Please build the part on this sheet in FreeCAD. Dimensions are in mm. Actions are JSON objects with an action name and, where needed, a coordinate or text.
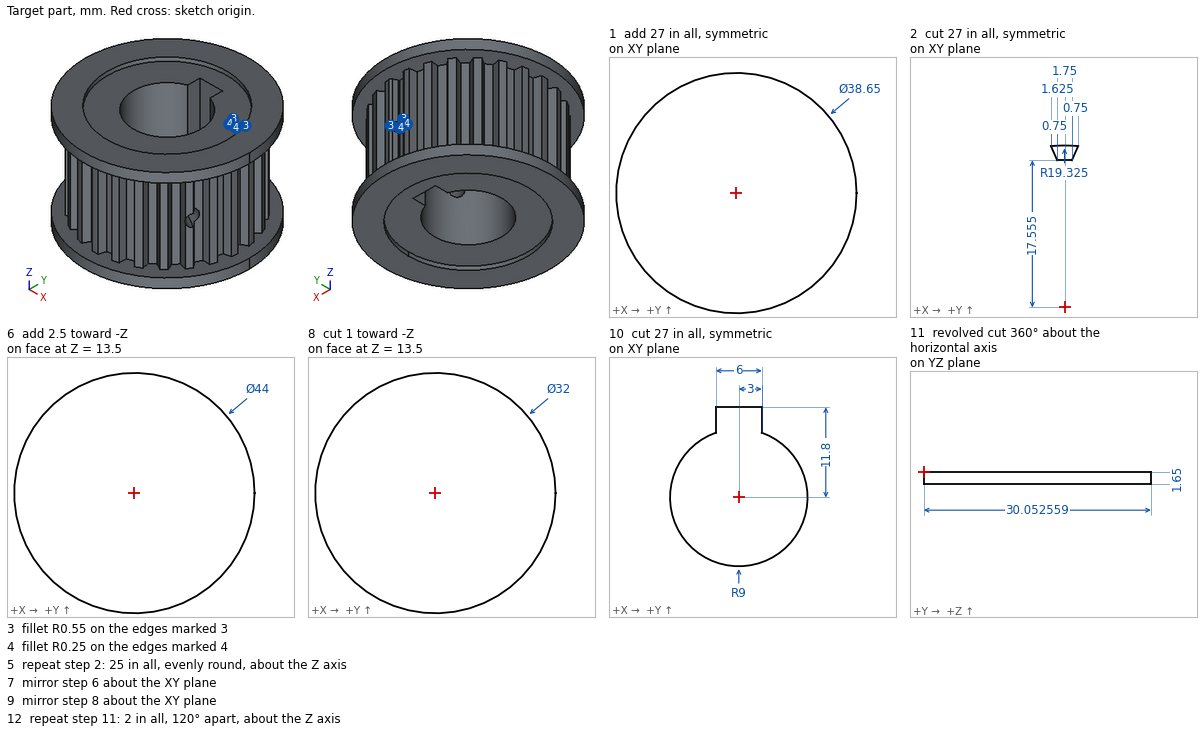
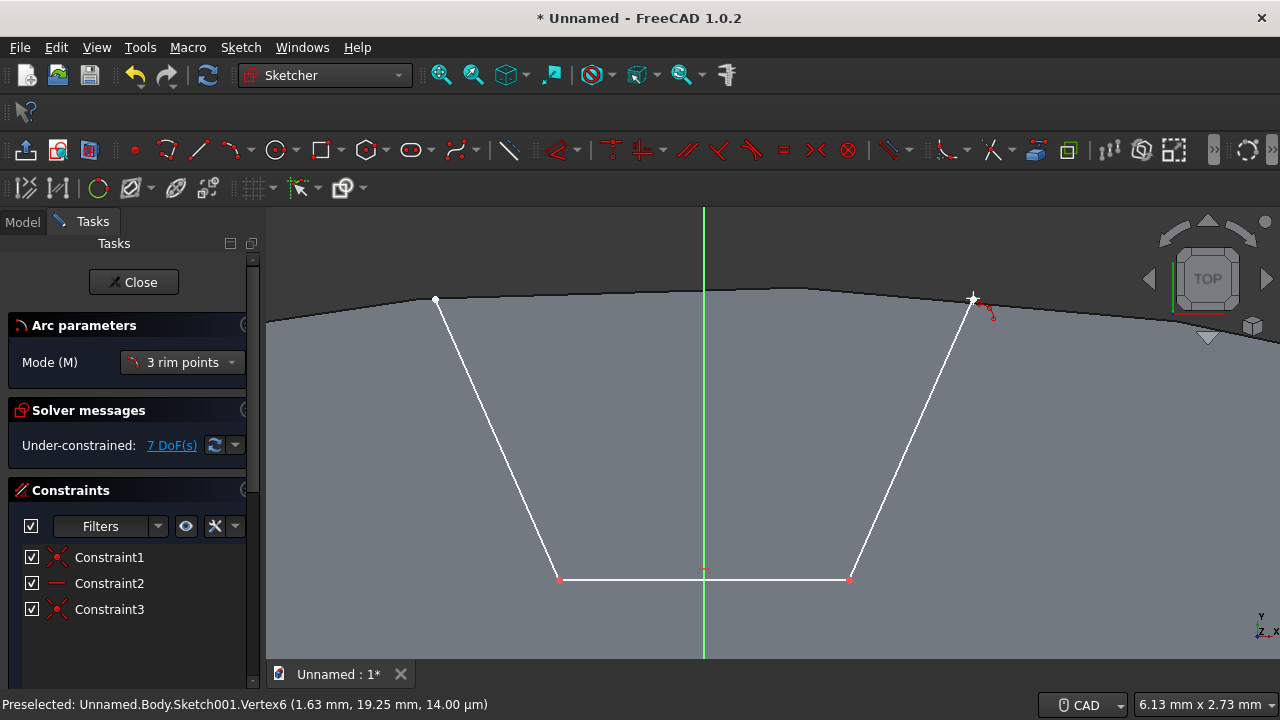
{"action": "left_click", "coordinate": [973, 299]}
{"action": "left_click", "coordinate": [435, 299]}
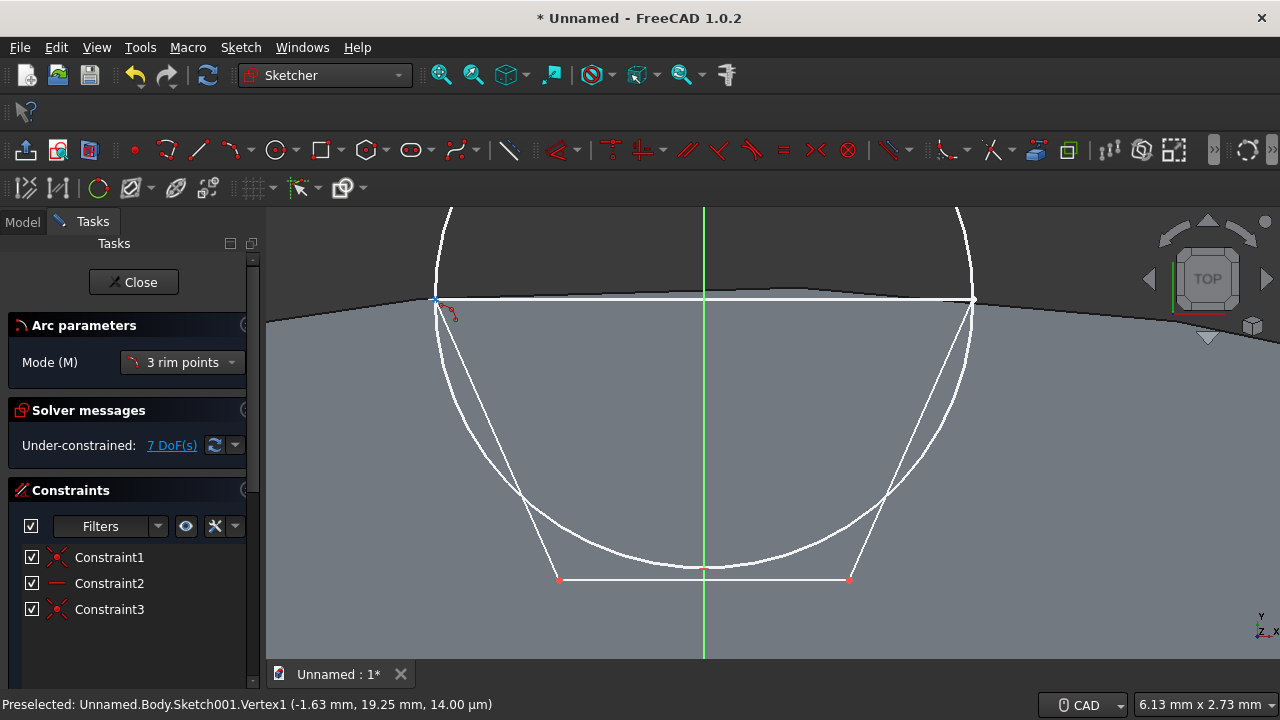
{"action": "scroll", "coordinate": [758, 287], "scroll_direction": "up", "scroll_amount": 2}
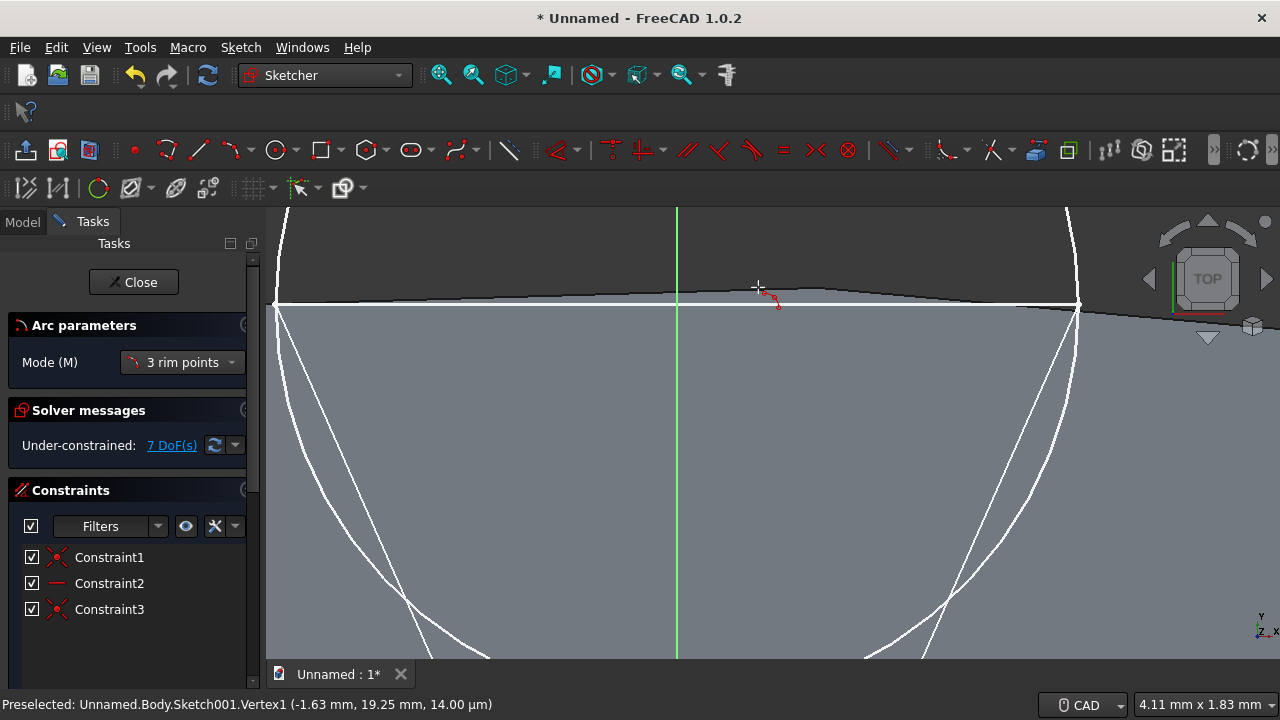
{"action": "left_click", "coordinate": [757, 286]}
{"action": "key", "text": "Escape"}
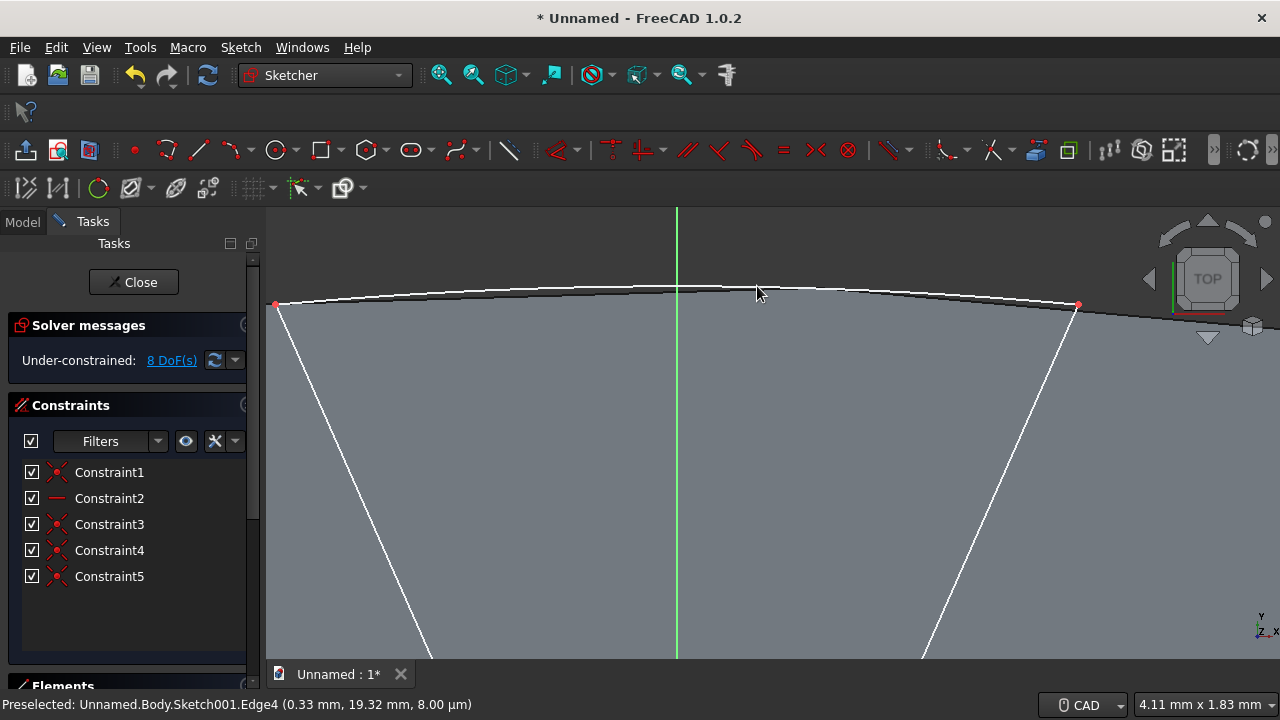
{"action": "scroll", "coordinate": [760, 288], "scroll_direction": "down", "scroll_amount": 2}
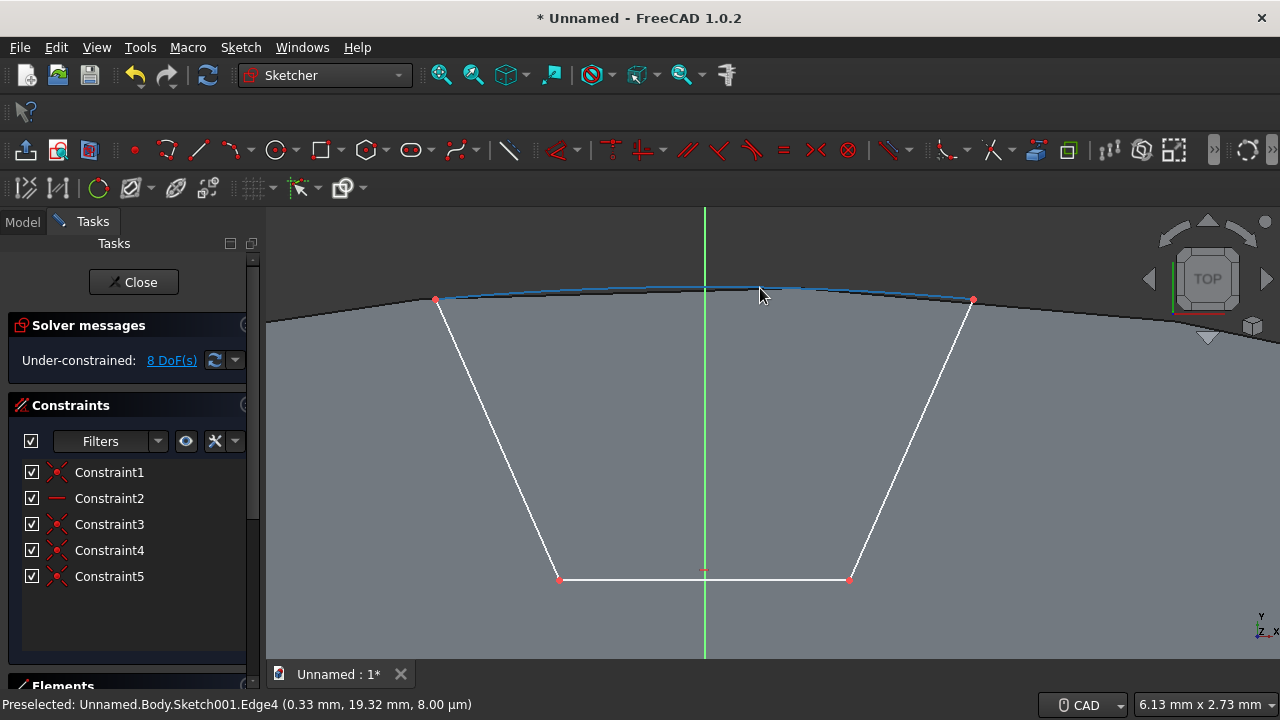
{"action": "scroll", "coordinate": [704, 295], "scroll_direction": "down", "scroll_amount": 12}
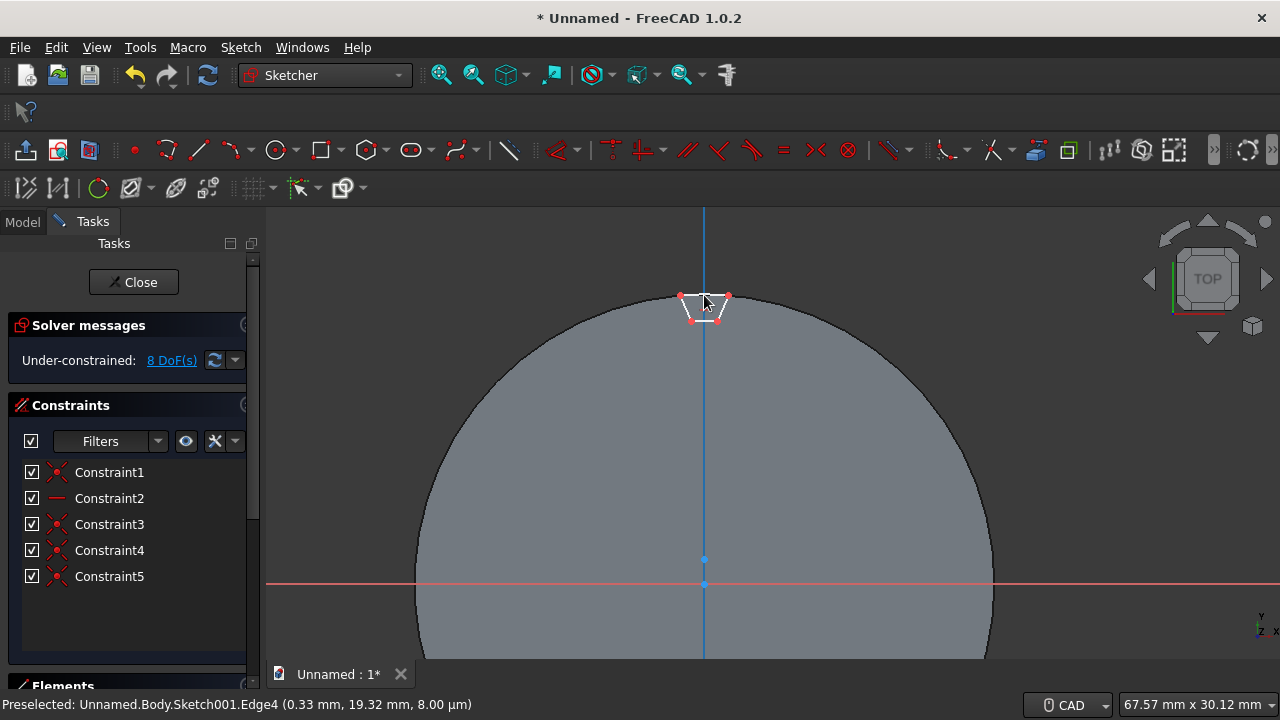
{"action": "left_click_drag", "start_coordinate": [694, 549], "coordinate": [714, 594]}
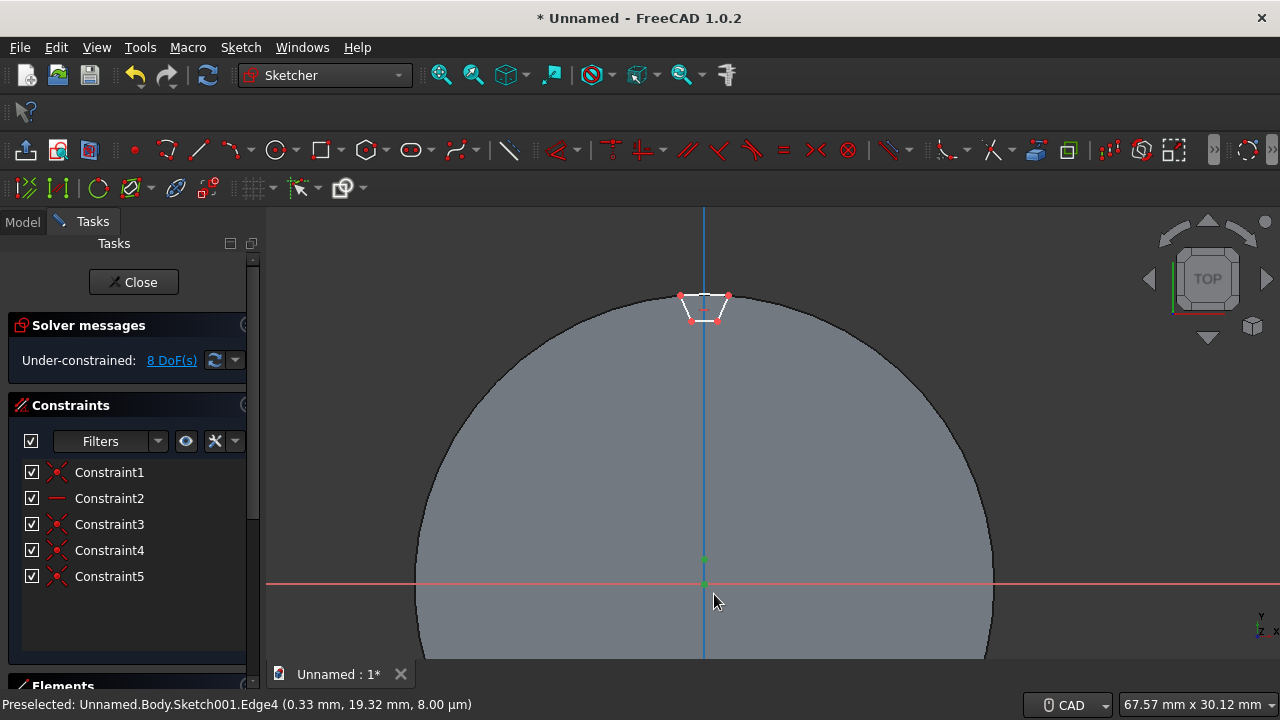
{"action": "left_click", "coordinate": [612, 150]}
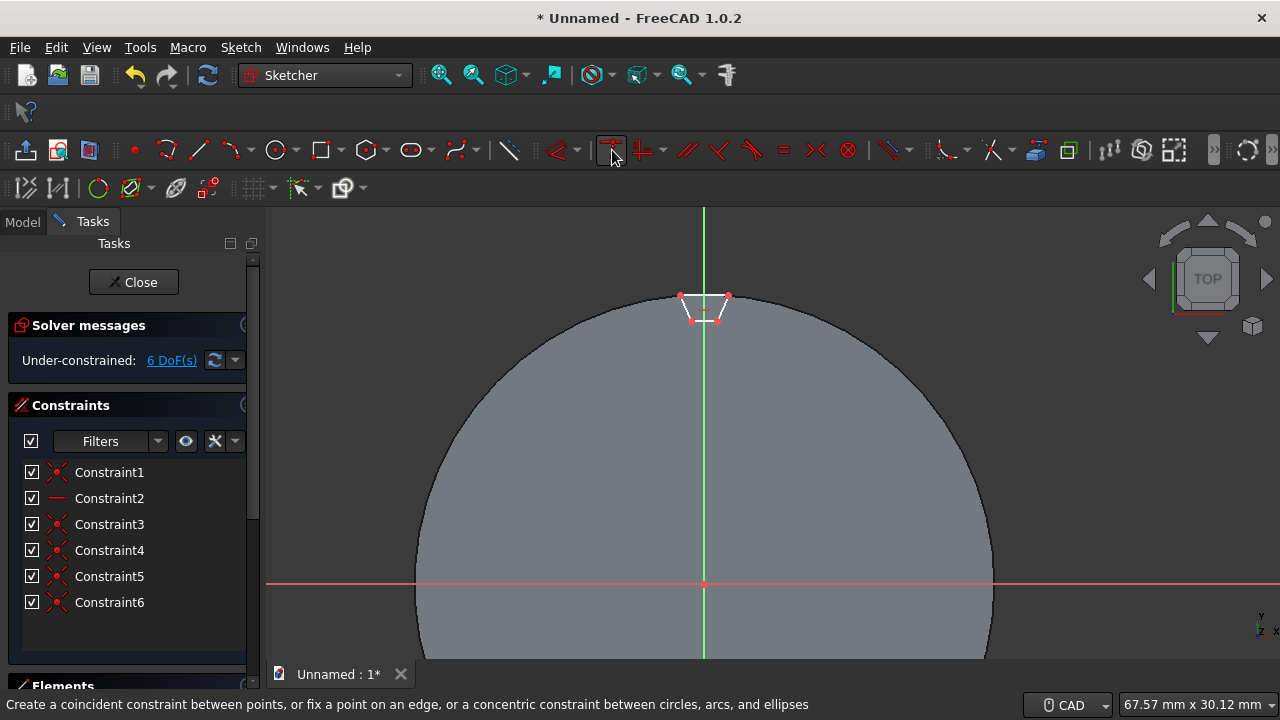
{"action": "scroll", "coordinate": [714, 295], "scroll_direction": "up", "scroll_amount": 2}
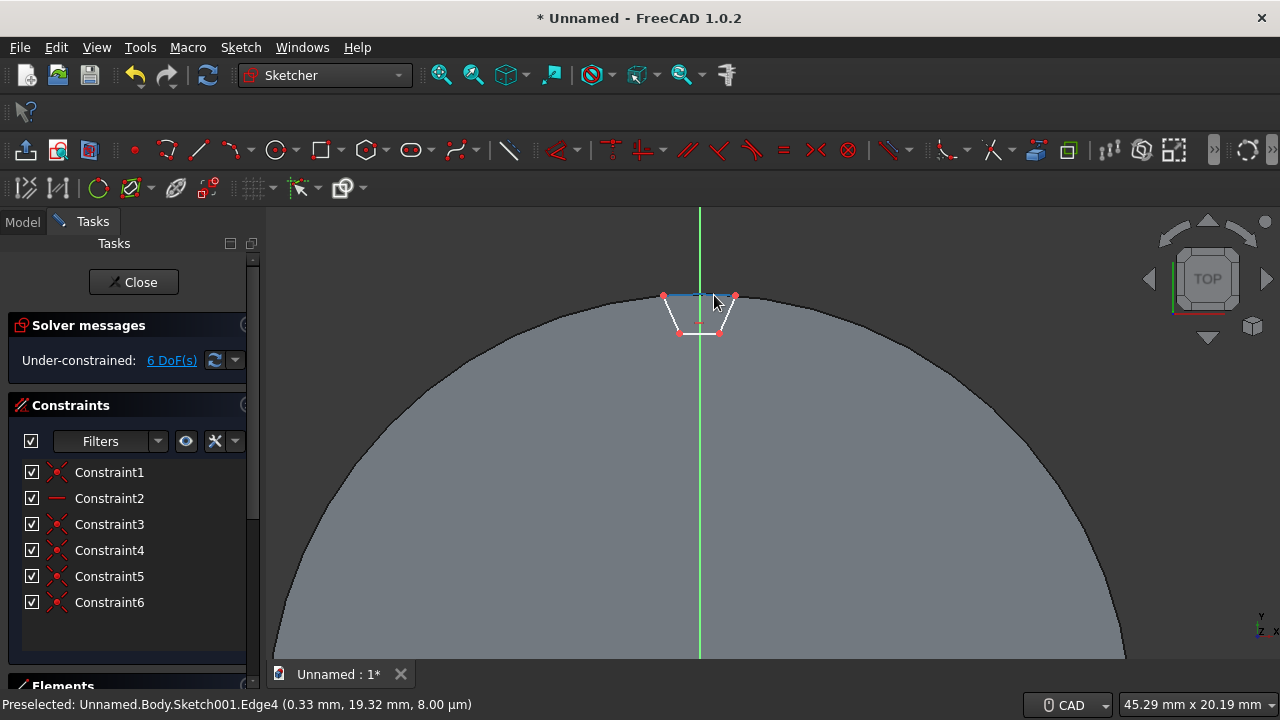
{"action": "left_click", "coordinate": [714, 295]}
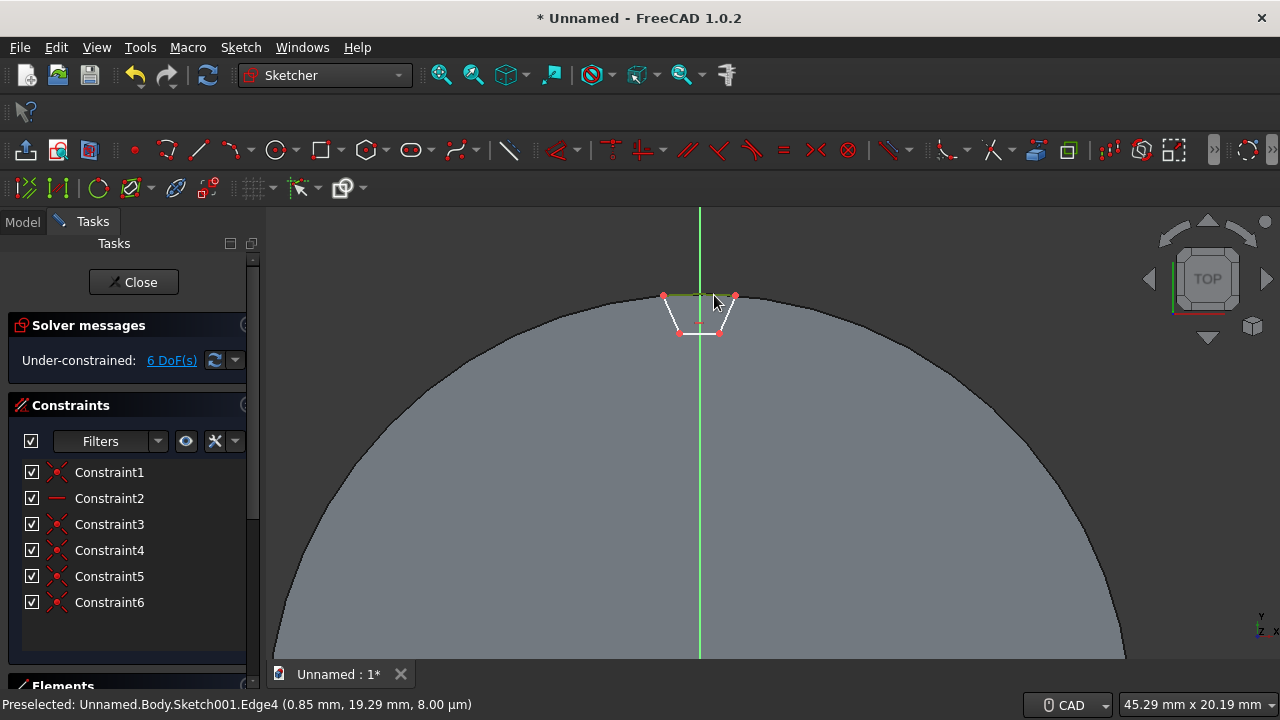
{"action": "left_click", "coordinate": [580, 150]}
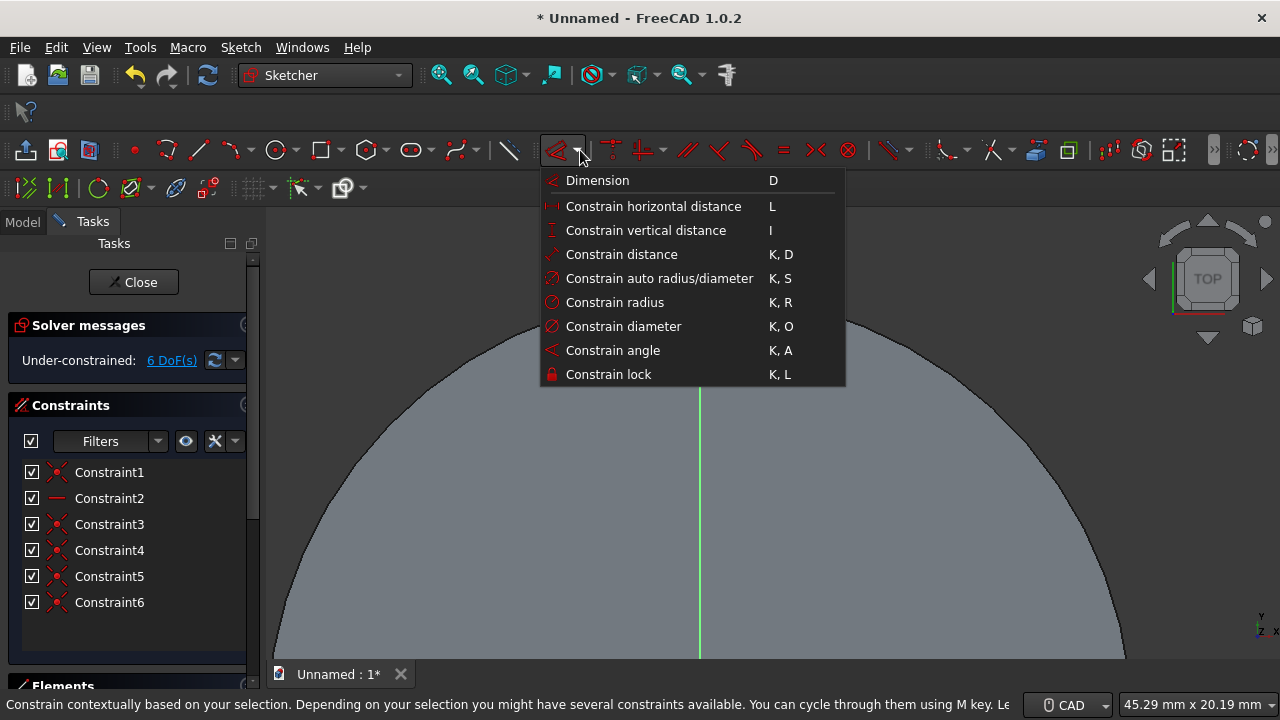
{"action": "left_click", "coordinate": [693, 302]}